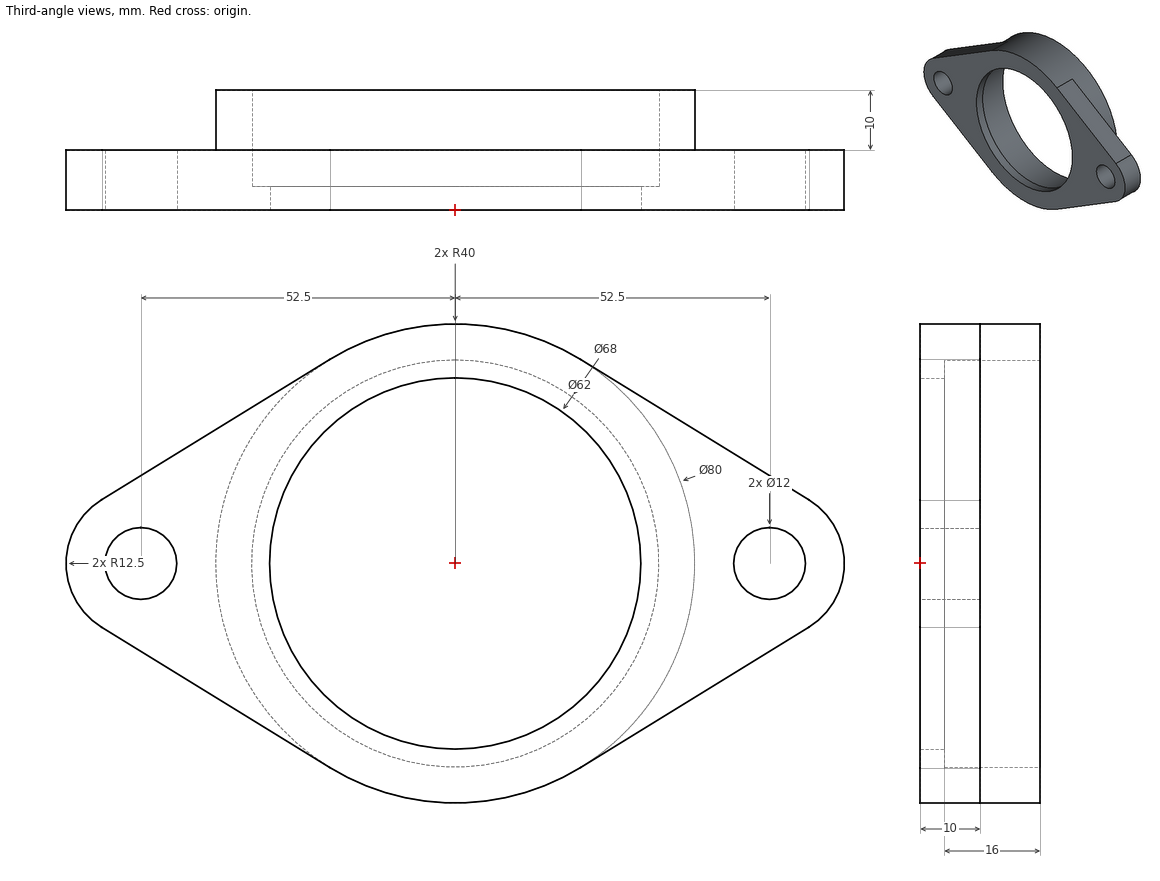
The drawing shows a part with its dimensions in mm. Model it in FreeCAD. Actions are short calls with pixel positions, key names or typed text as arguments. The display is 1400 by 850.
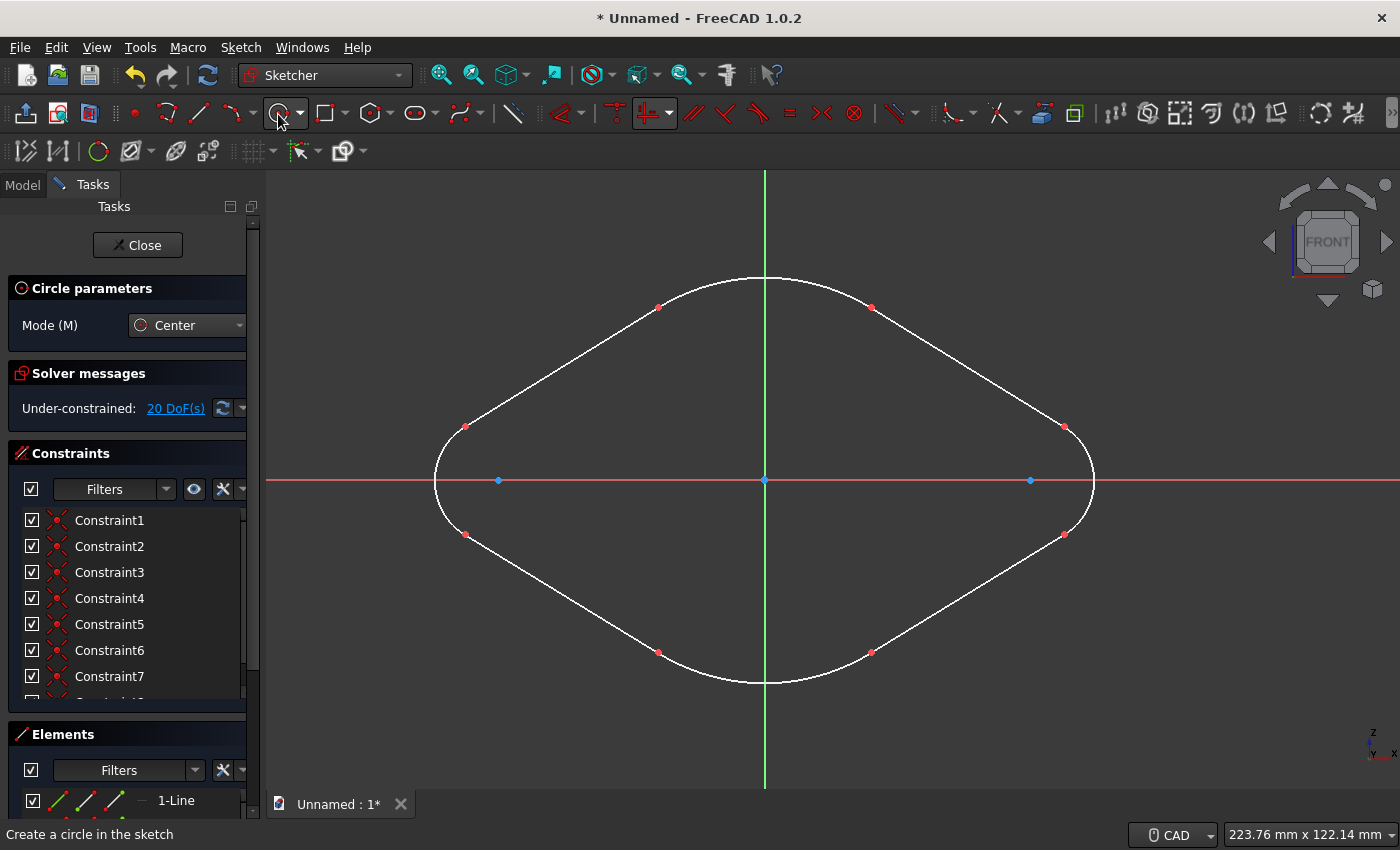
click(1031, 480)
move(1052, 458)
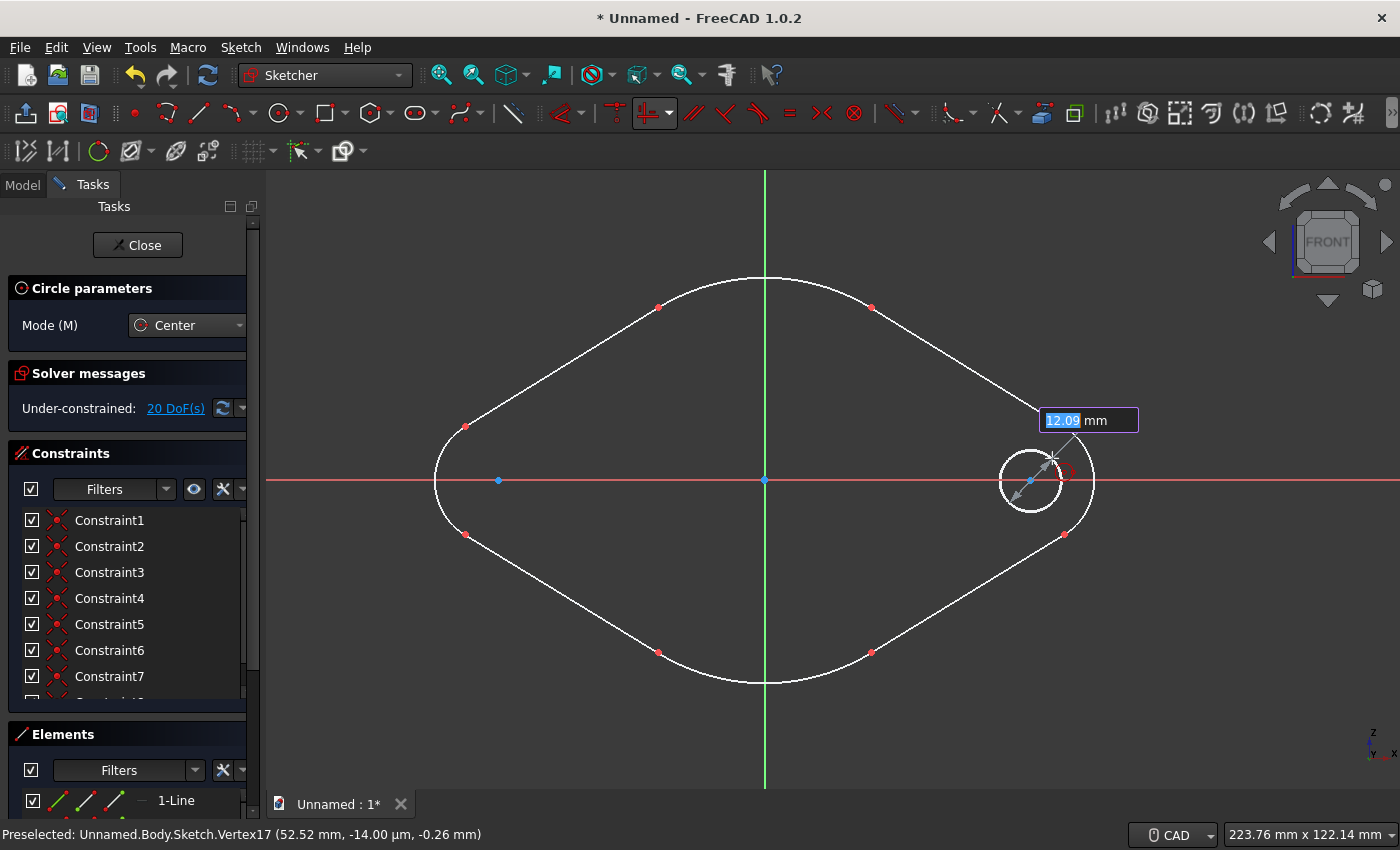
text(12)
key(Return)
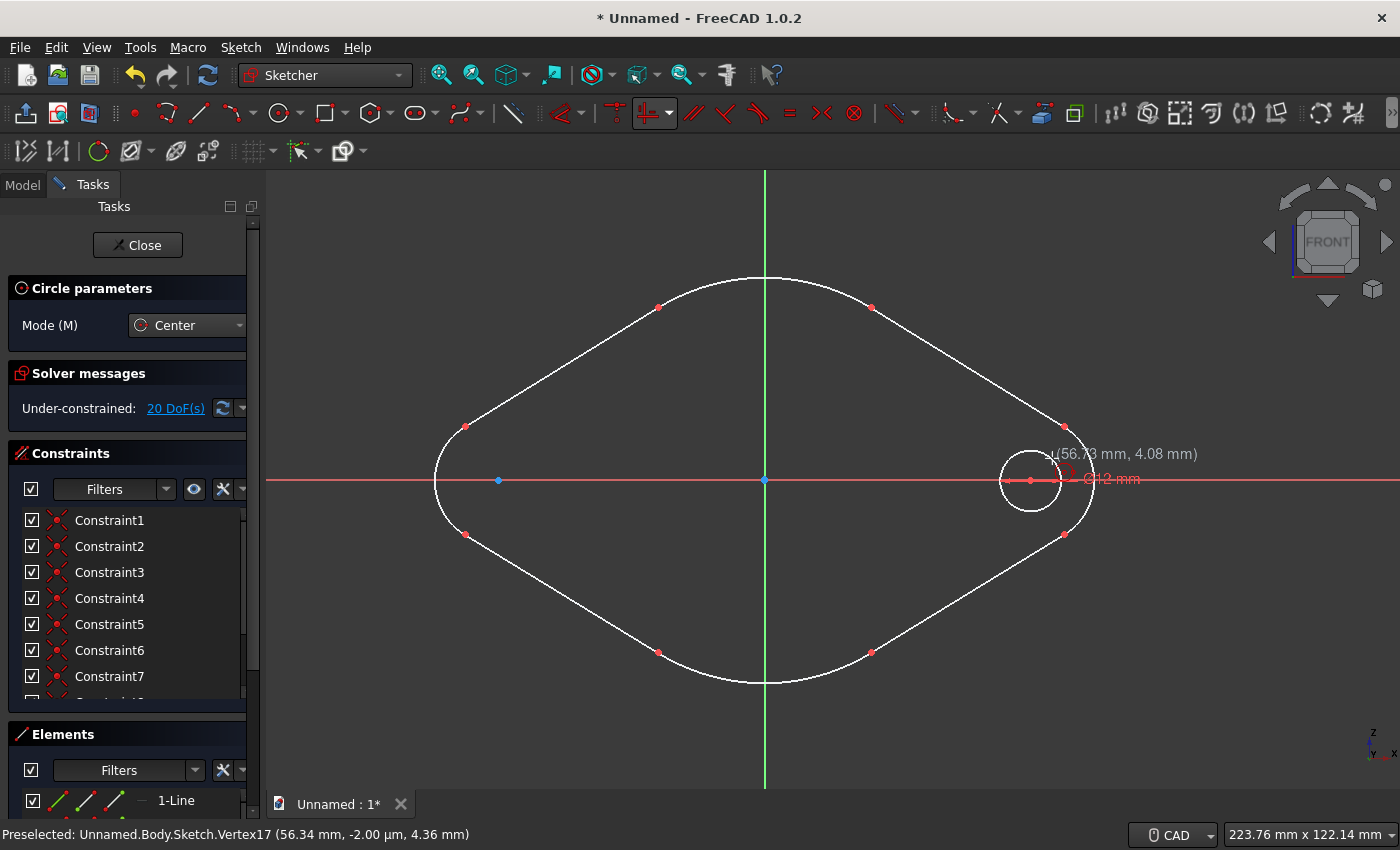
click(498, 480)
move(520, 458)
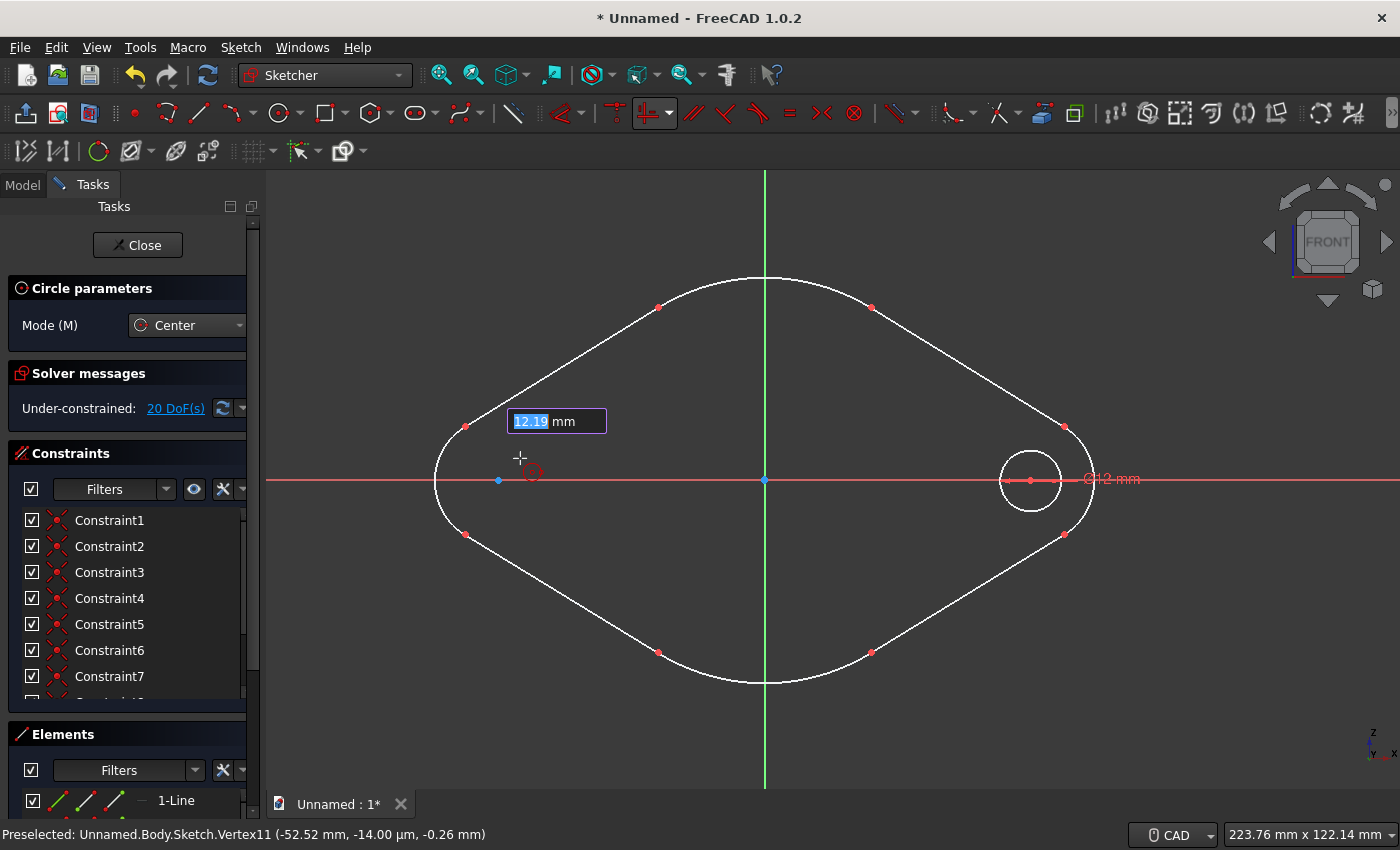
text(12)
key(Return)
key(Escape)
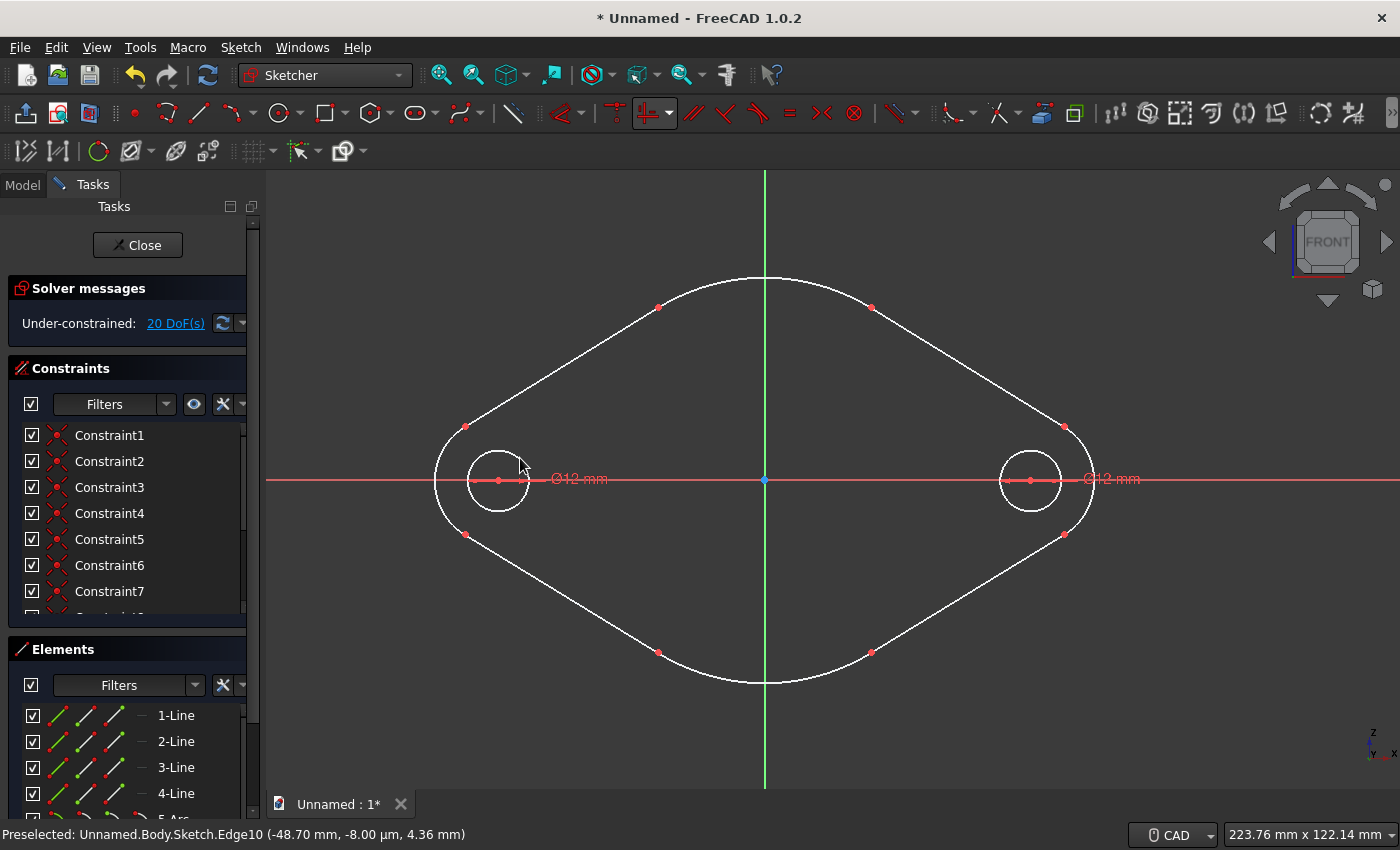
click(600, 618)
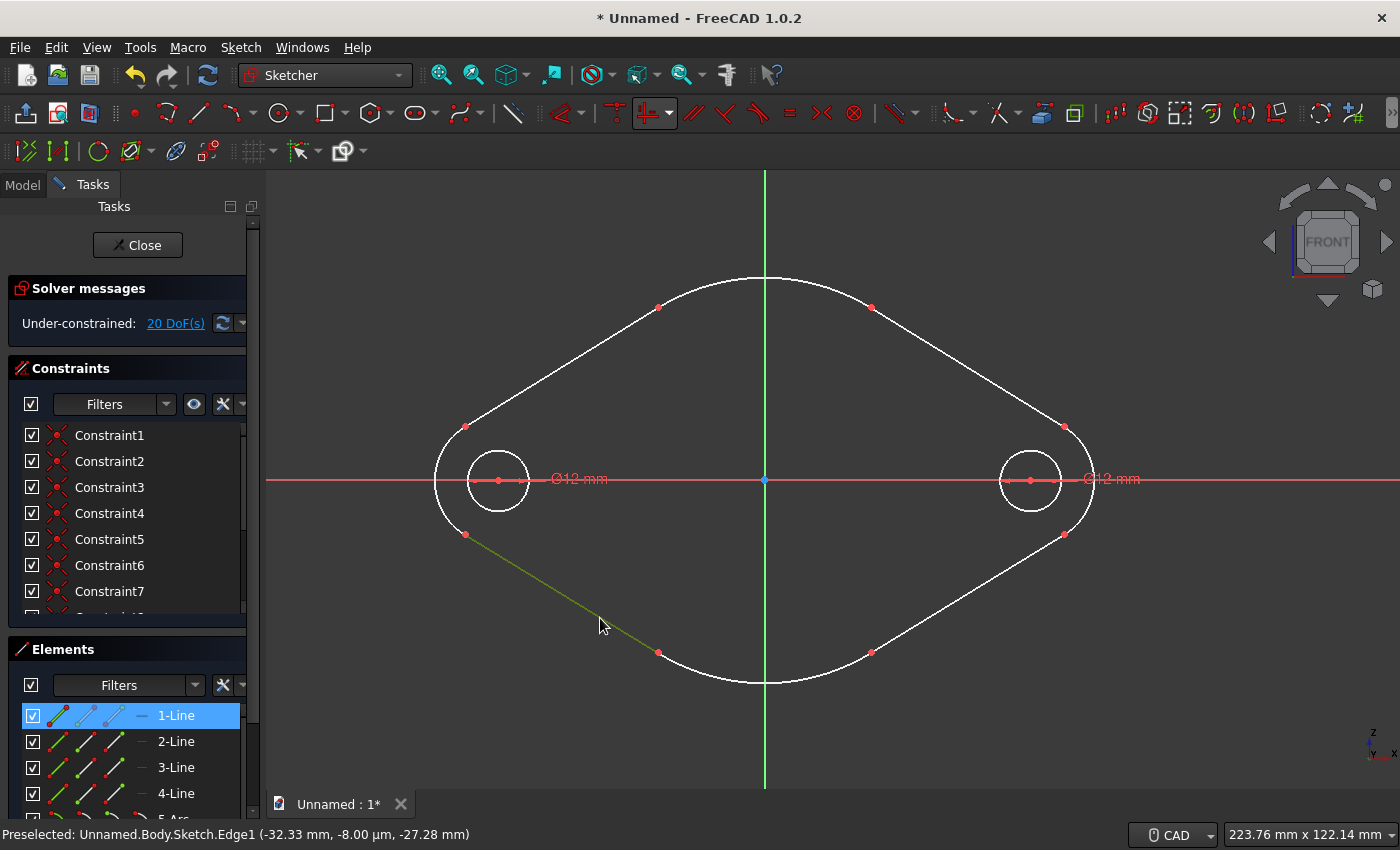
click(440, 456)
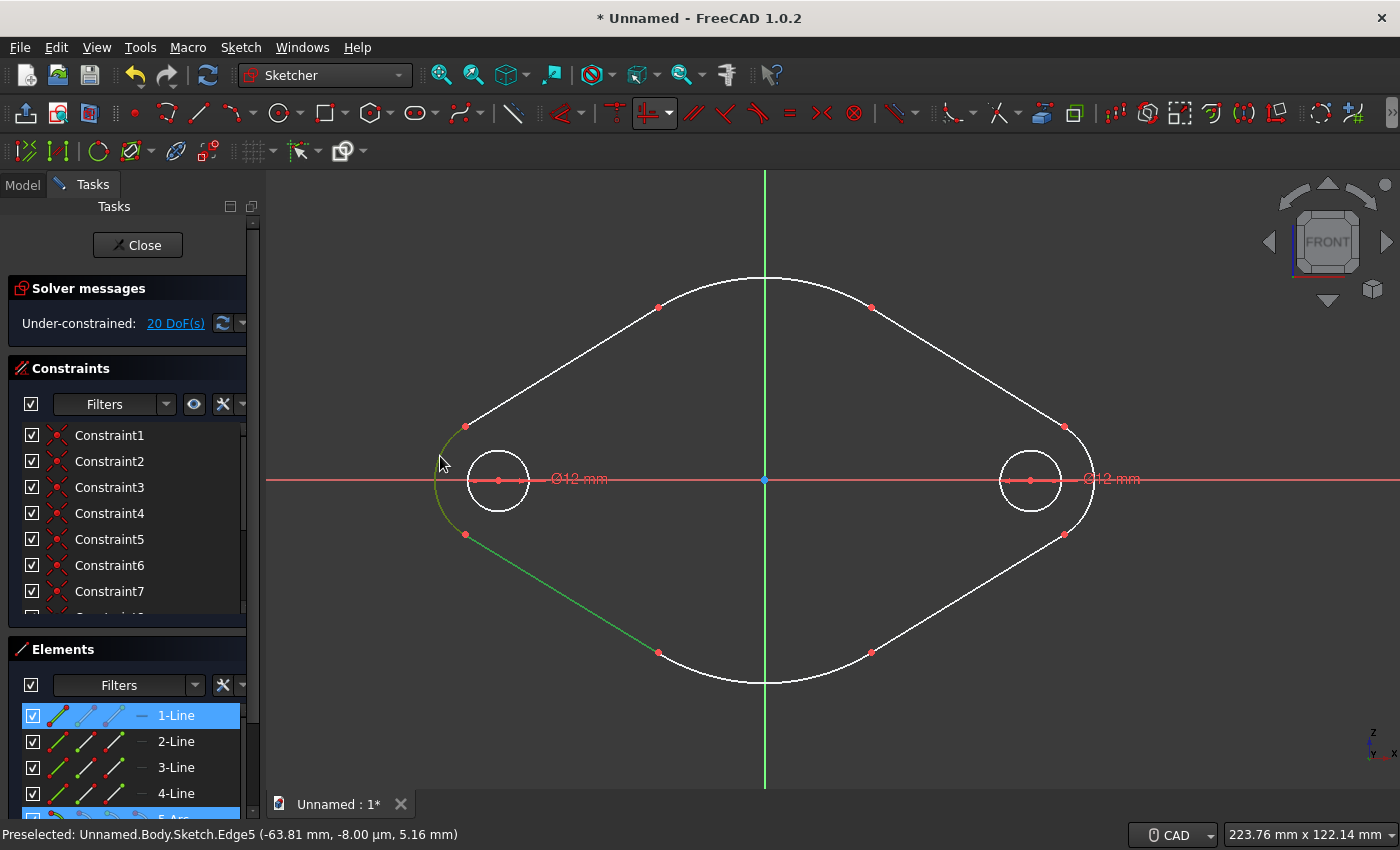
click(758, 114)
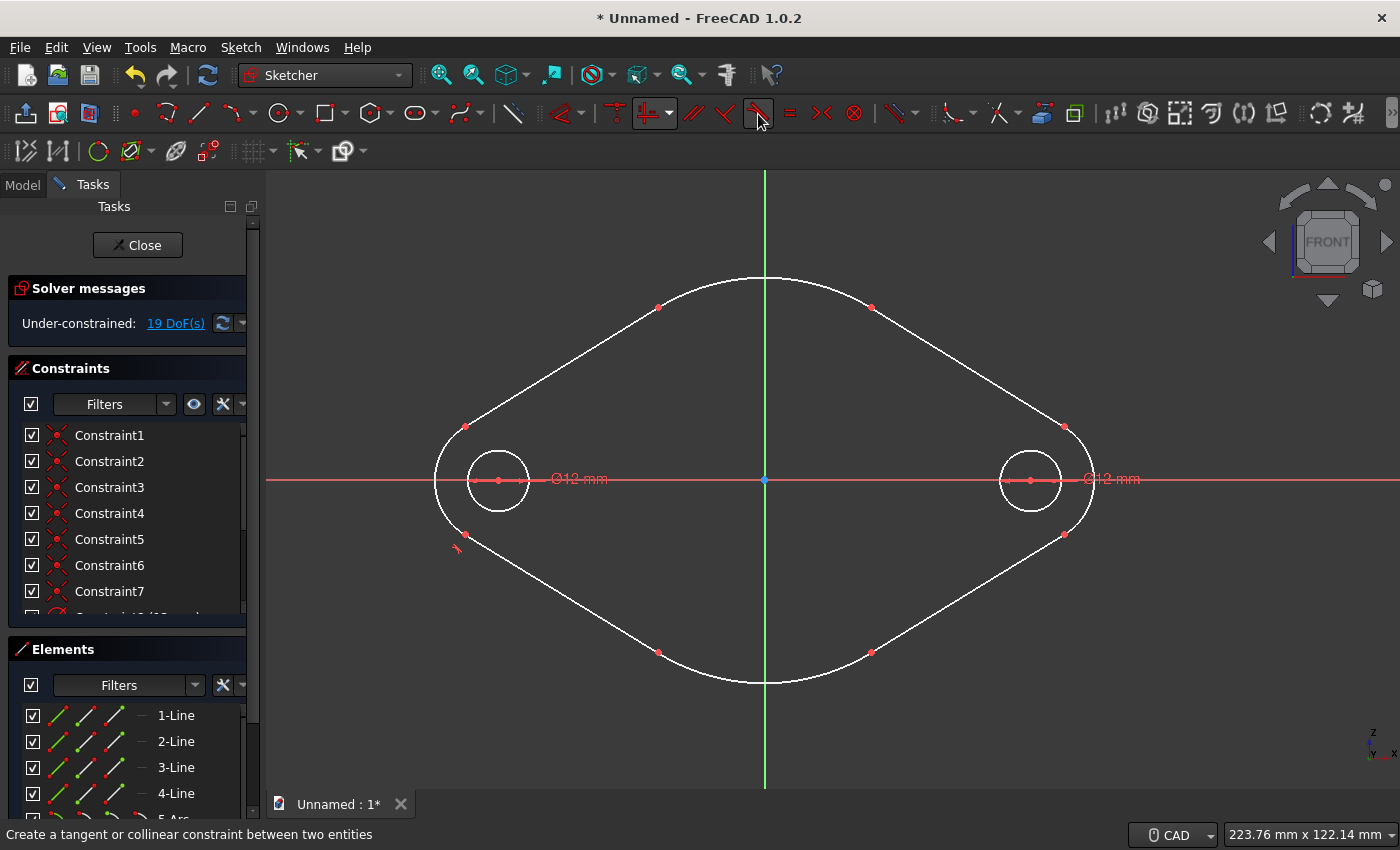
click(600, 618)